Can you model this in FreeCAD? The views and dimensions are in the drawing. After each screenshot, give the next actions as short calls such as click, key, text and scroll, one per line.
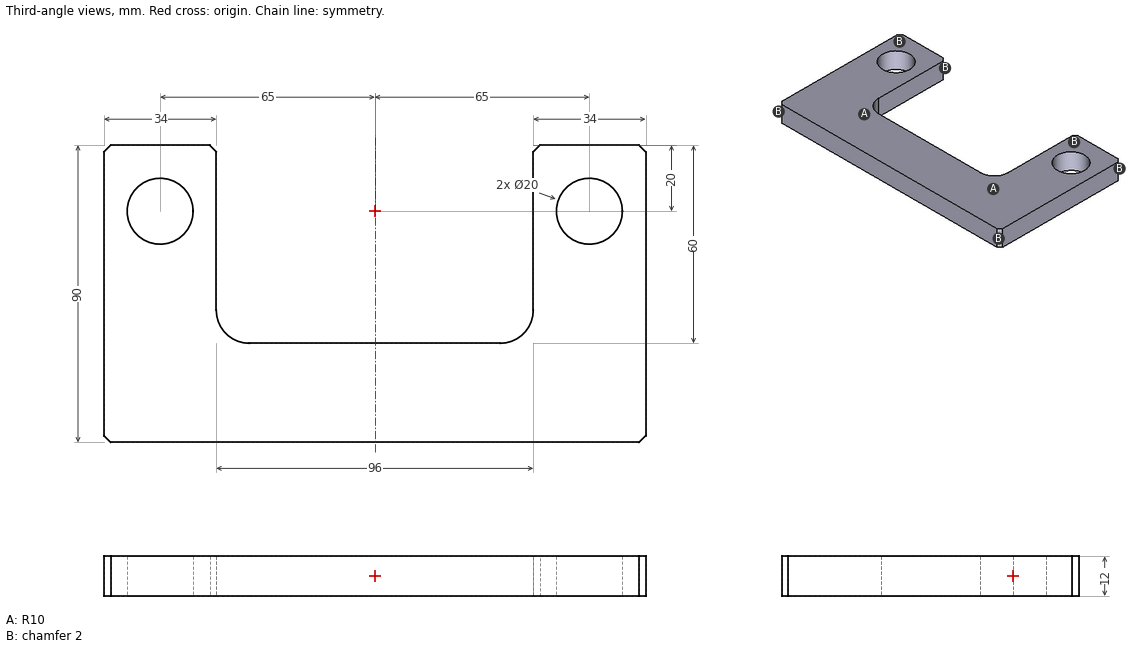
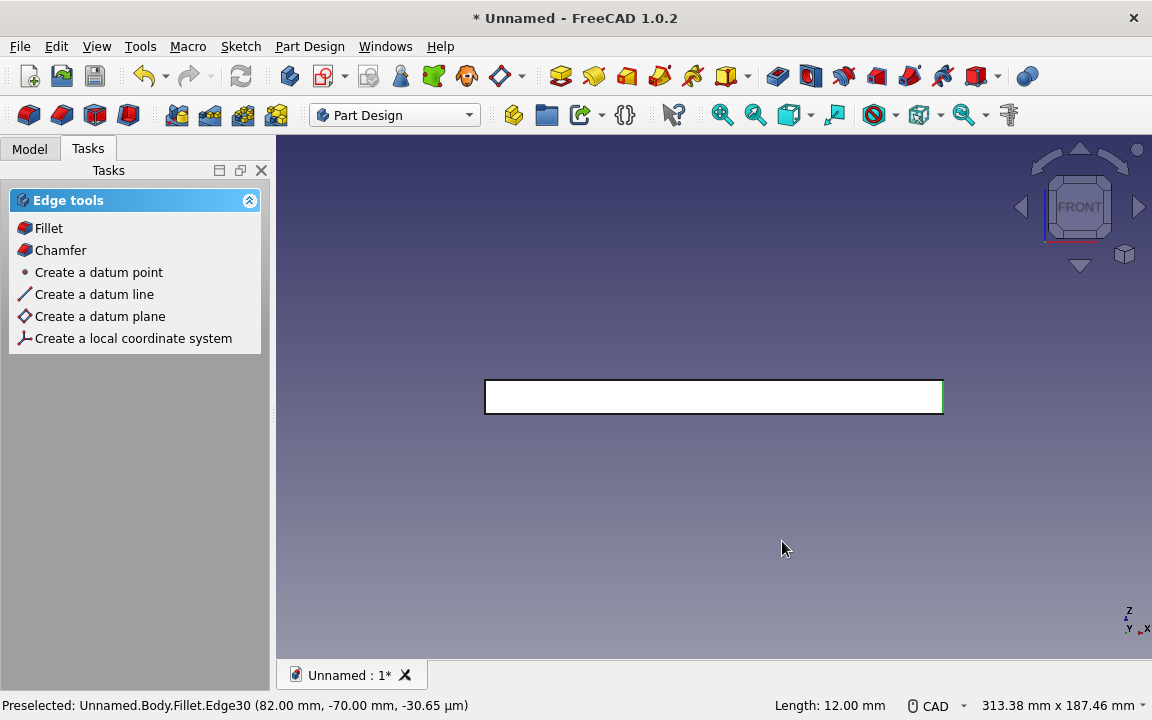
click(485, 396, ctrl)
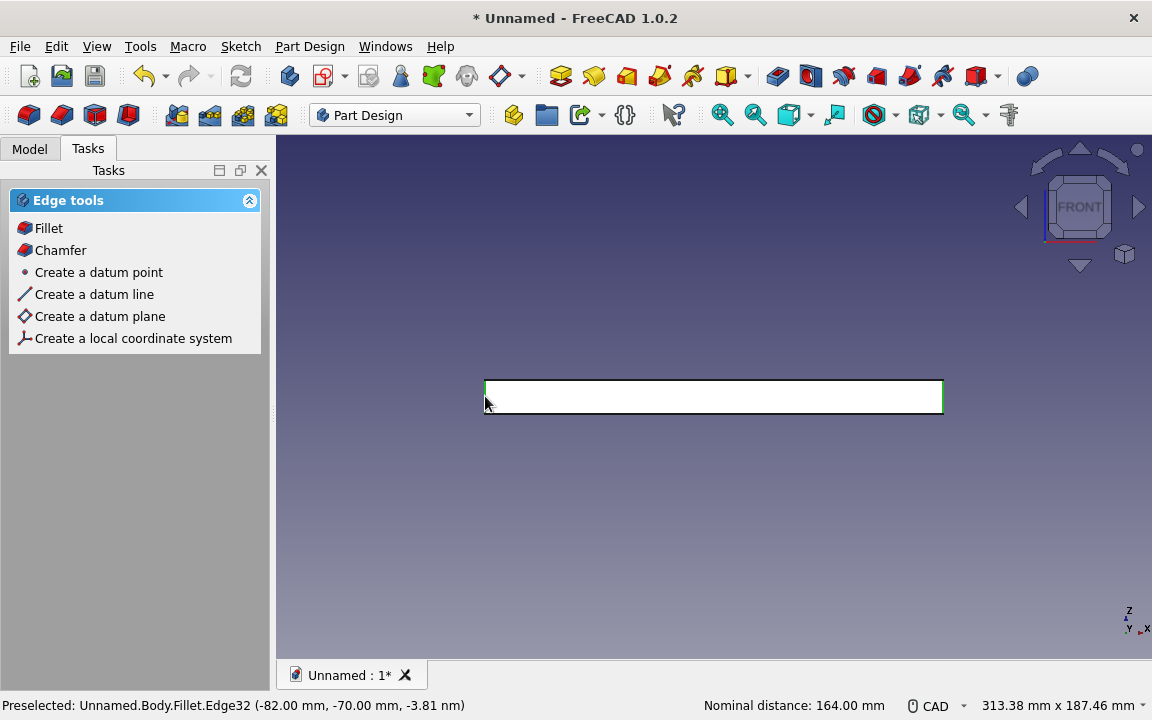
key(3)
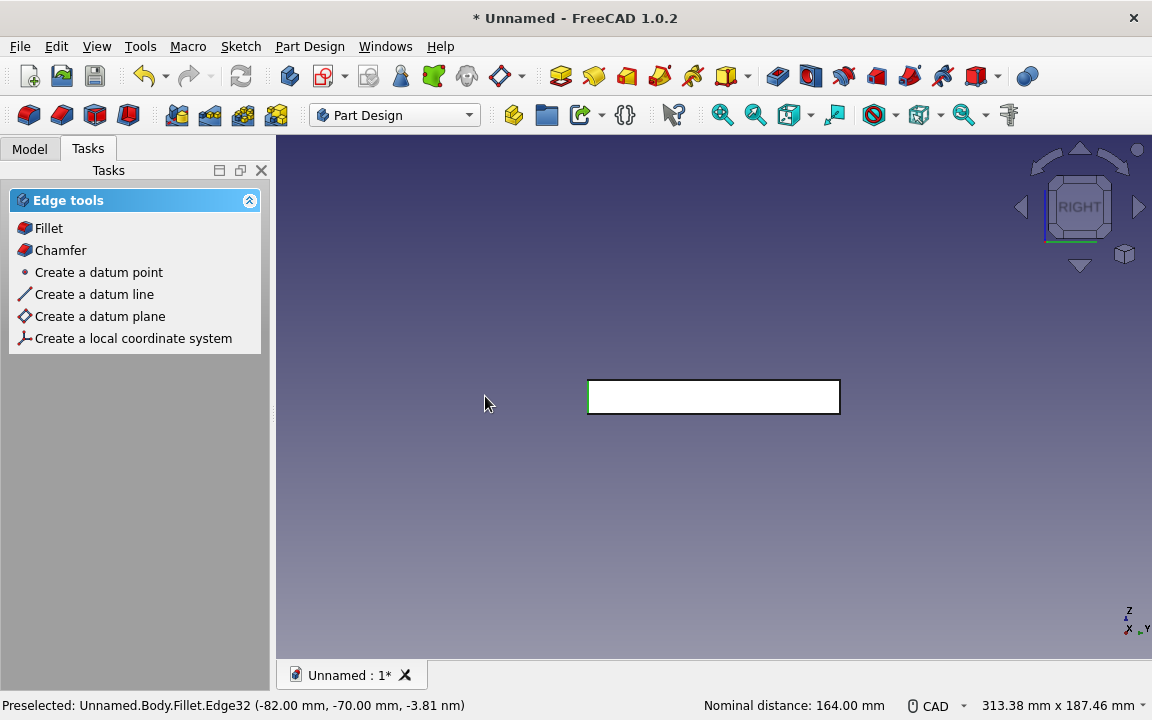
click(723, 116)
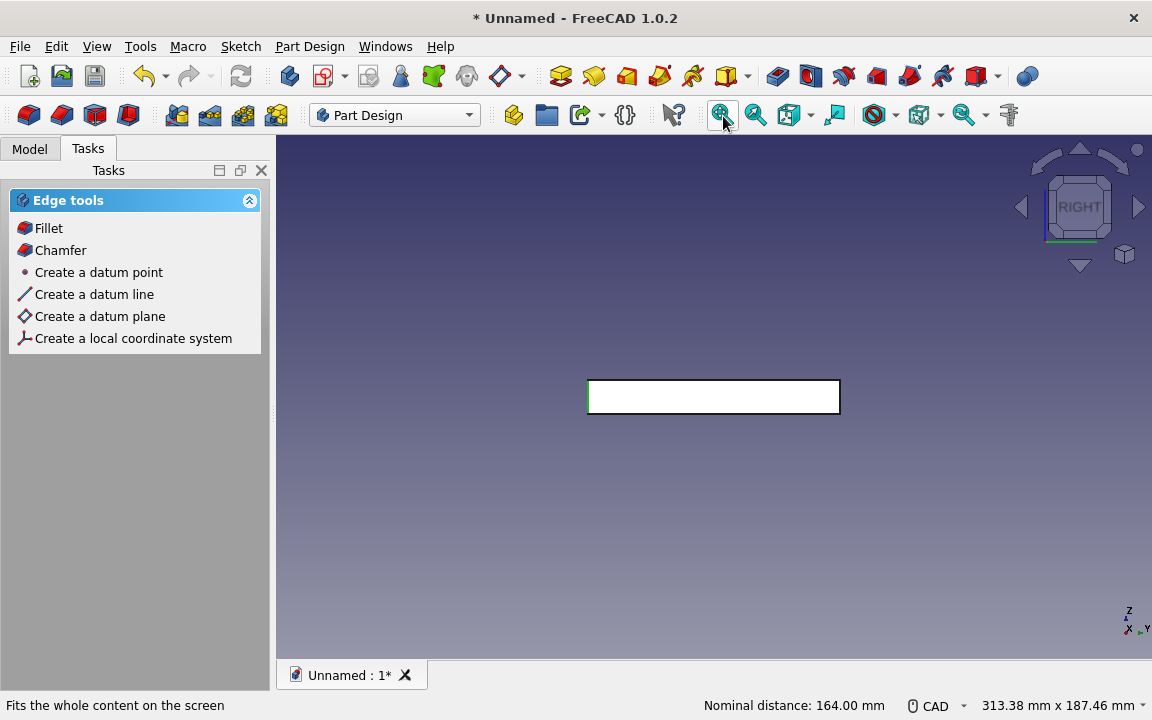
click(840, 396, ctrl)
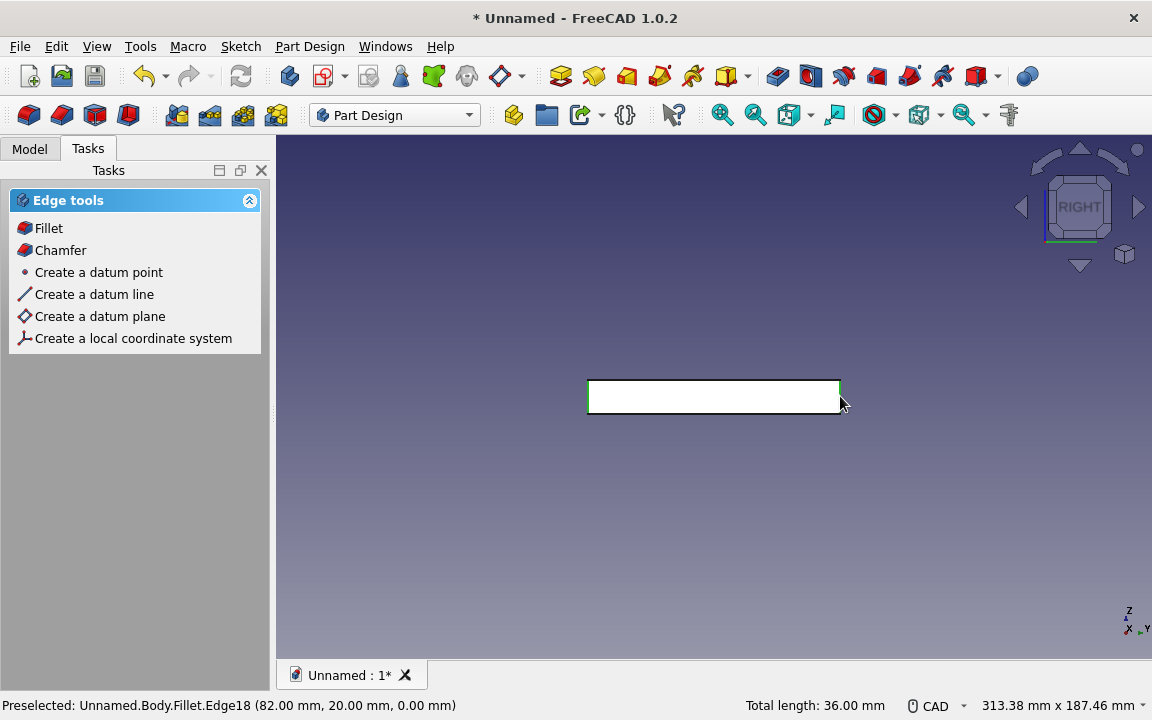
key(5)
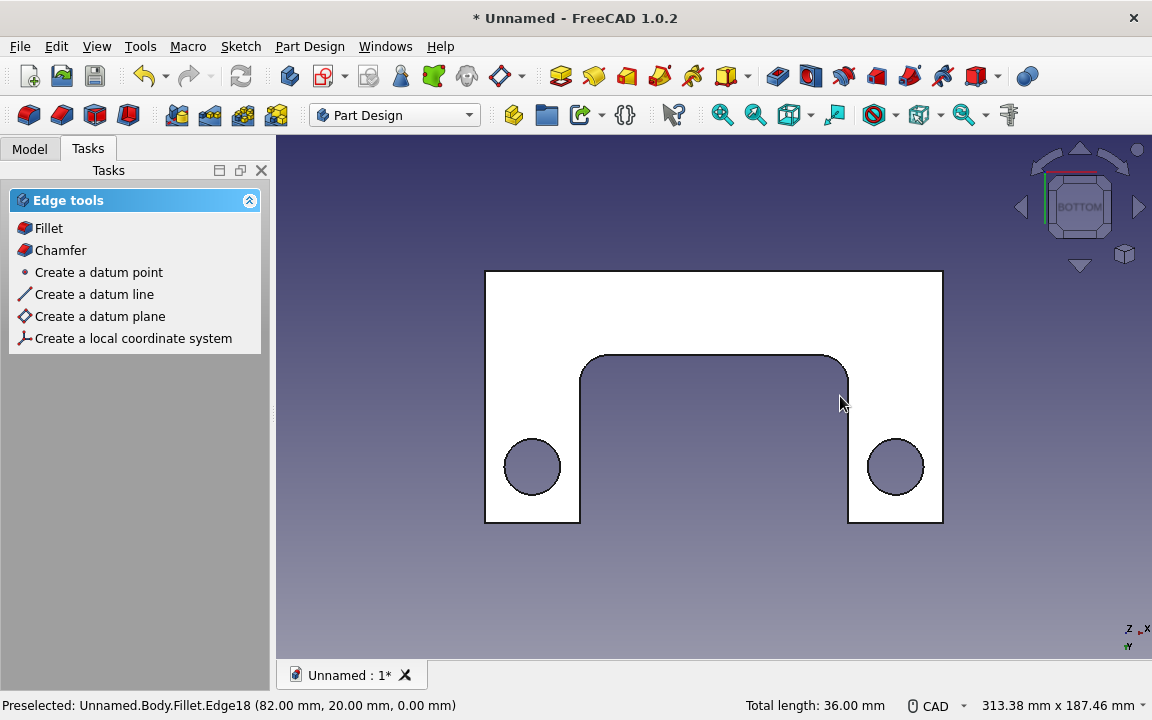
key(4)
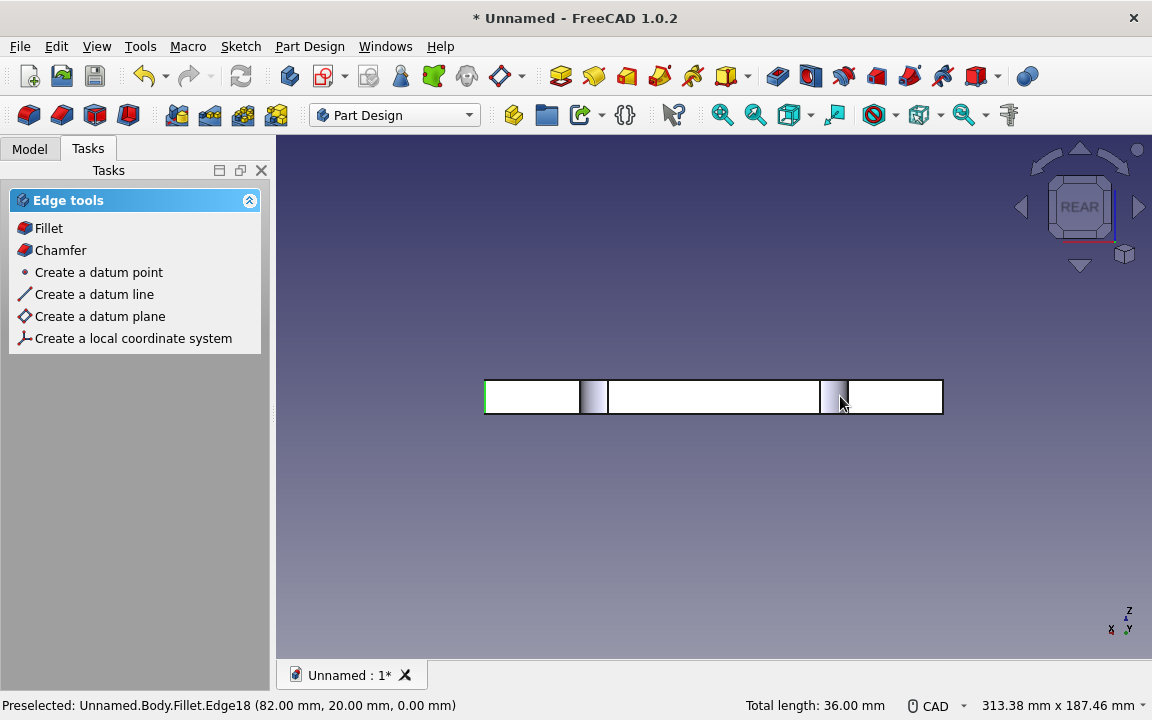
click(848, 396, ctrl)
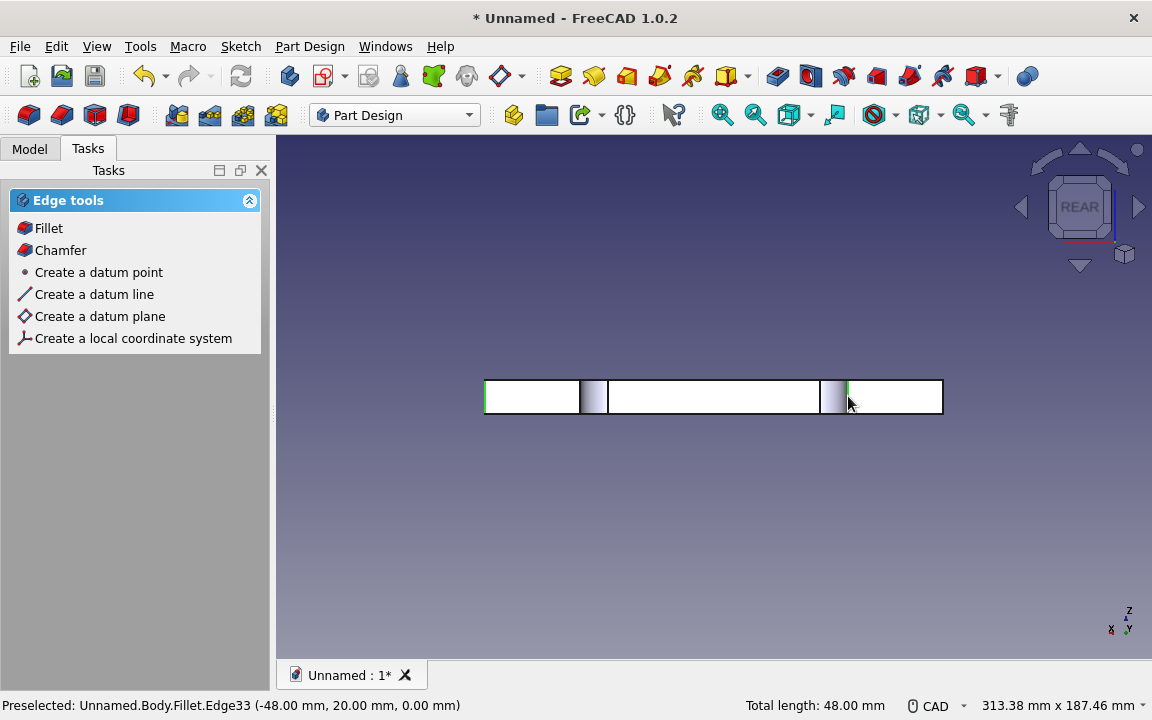
click(580, 396, ctrl)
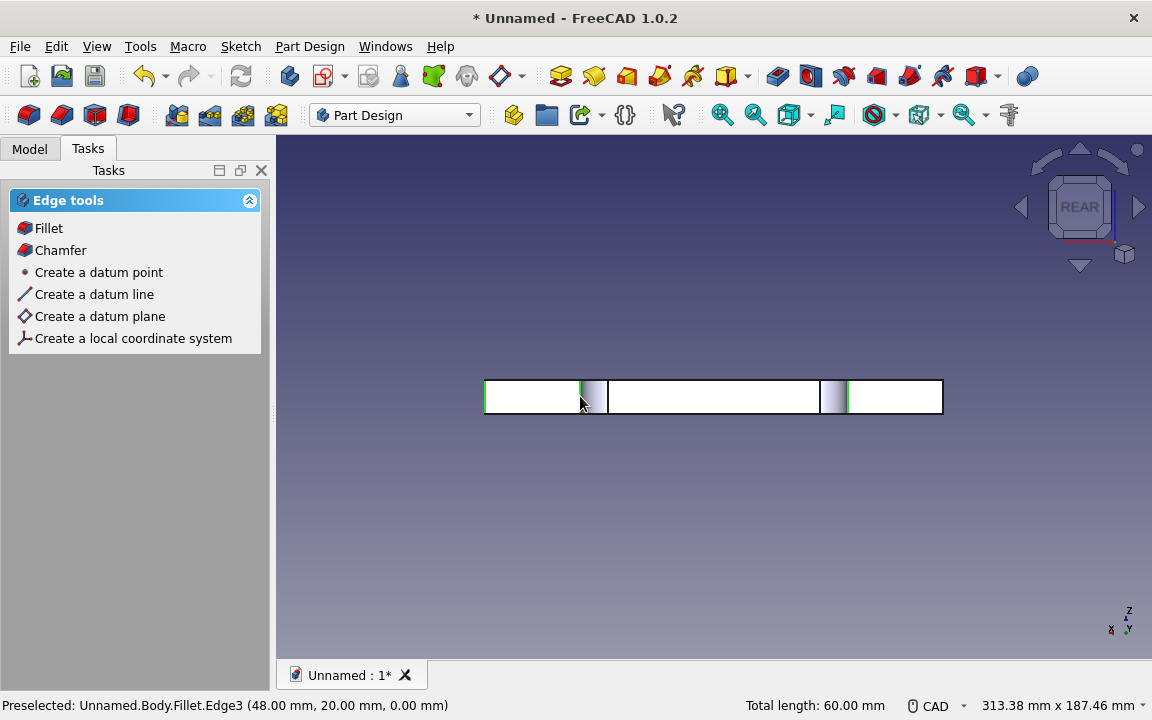
click(943, 396, ctrl)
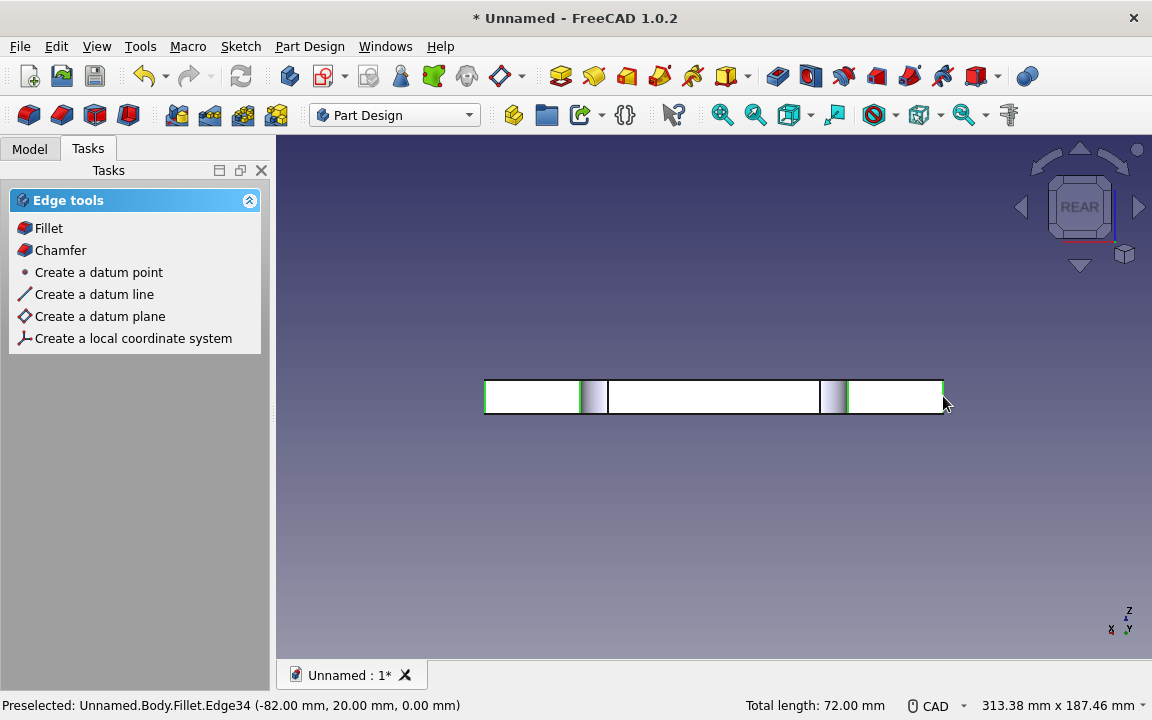
click(62, 116)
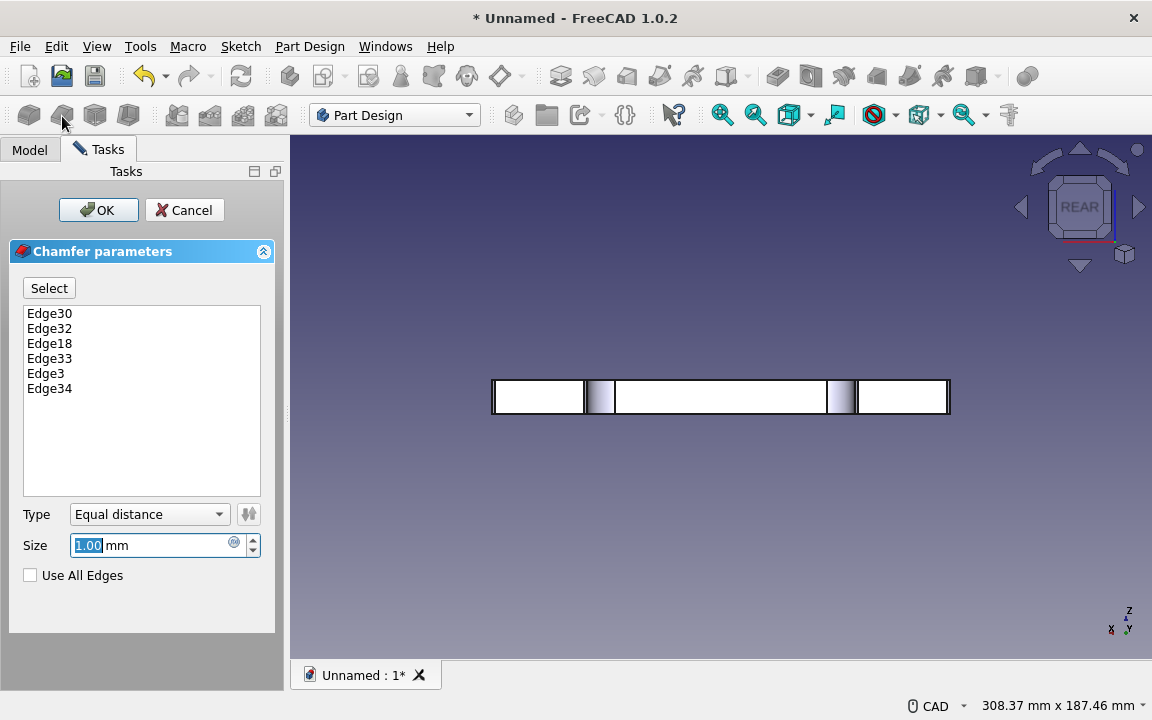
text(2)
key(Tab)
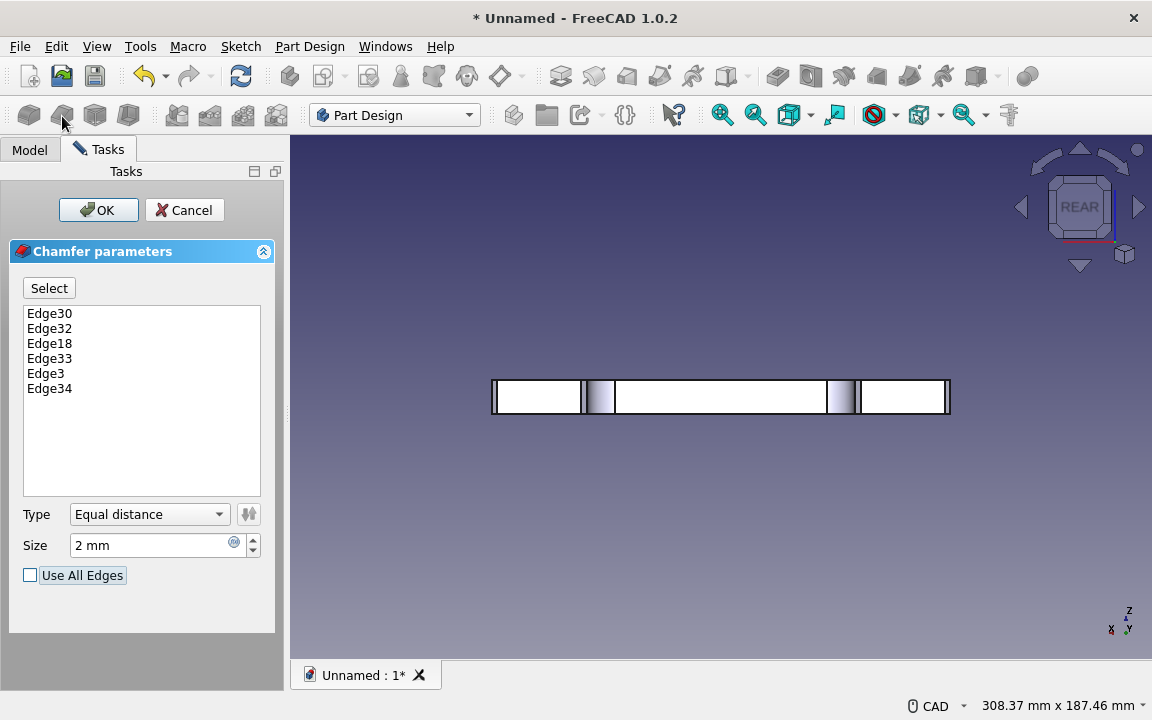
click(99, 210)